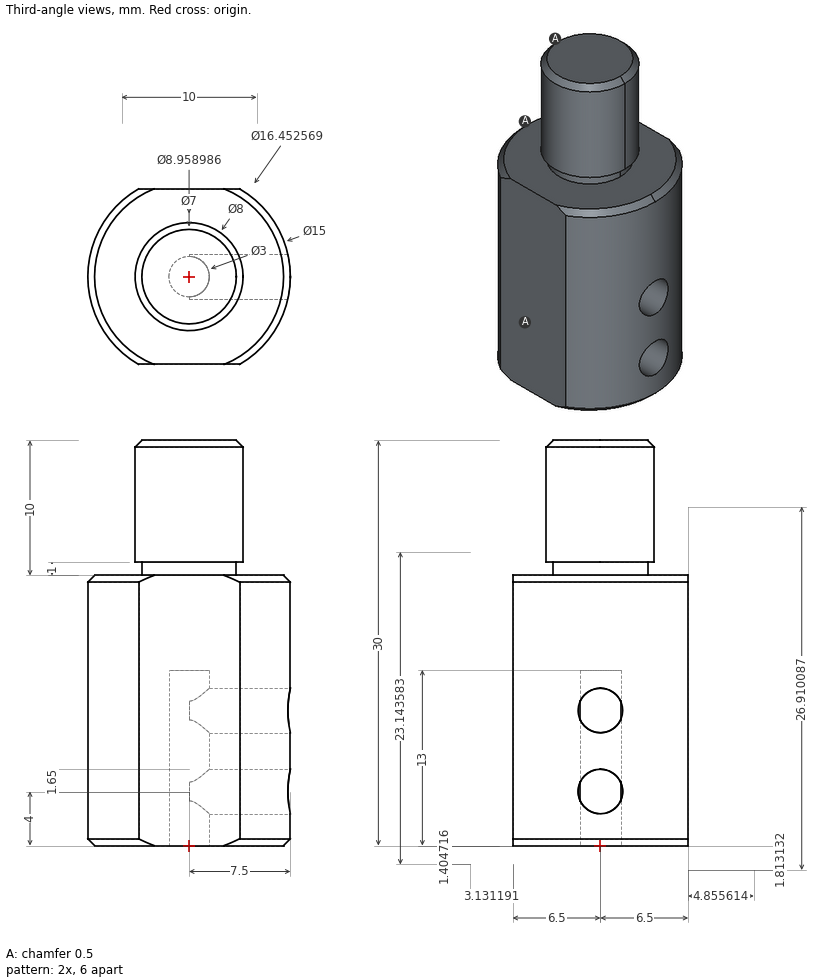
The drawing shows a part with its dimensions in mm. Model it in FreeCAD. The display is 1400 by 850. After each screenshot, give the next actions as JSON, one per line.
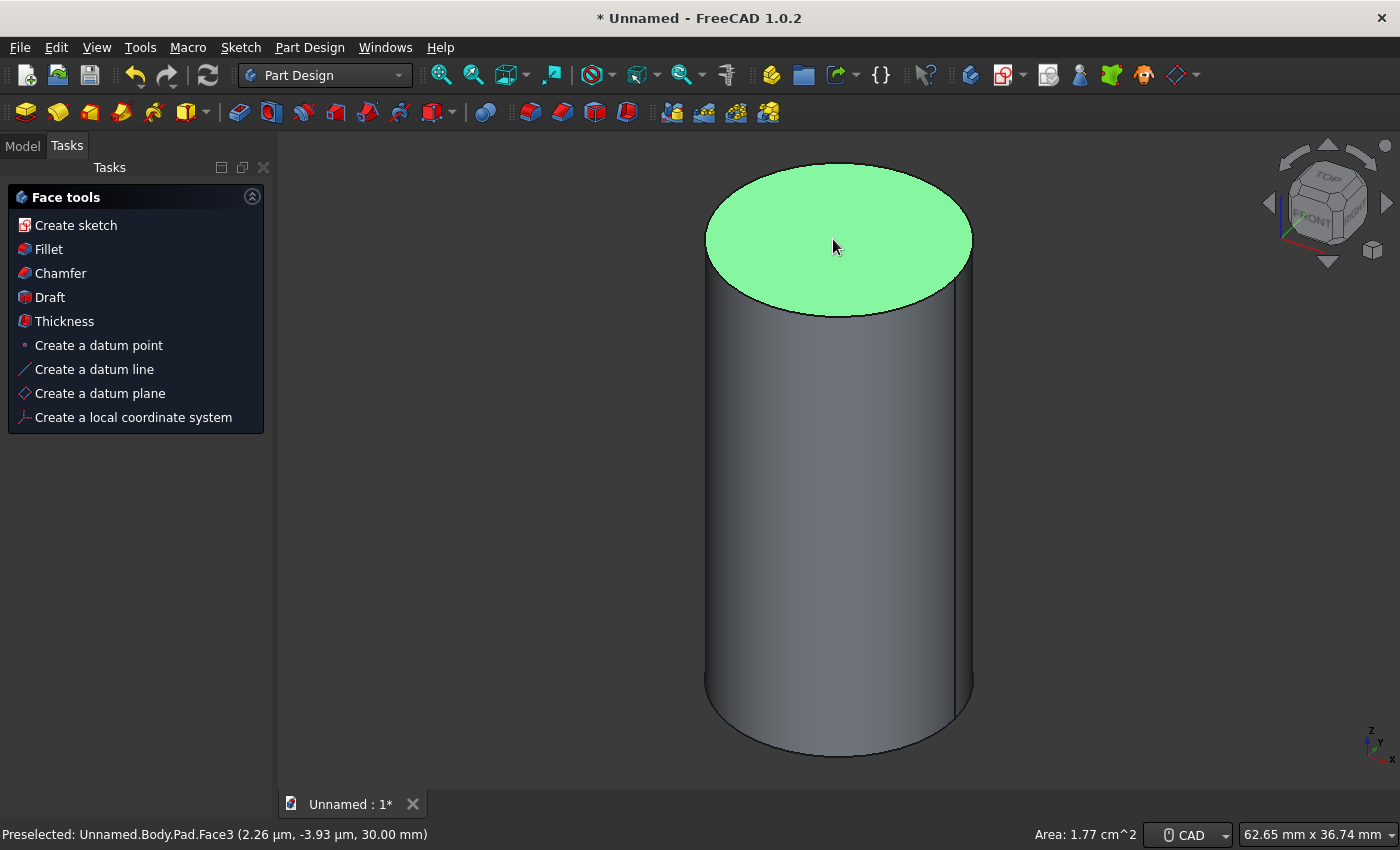
{"action": "left_click", "coordinate": [1004, 76]}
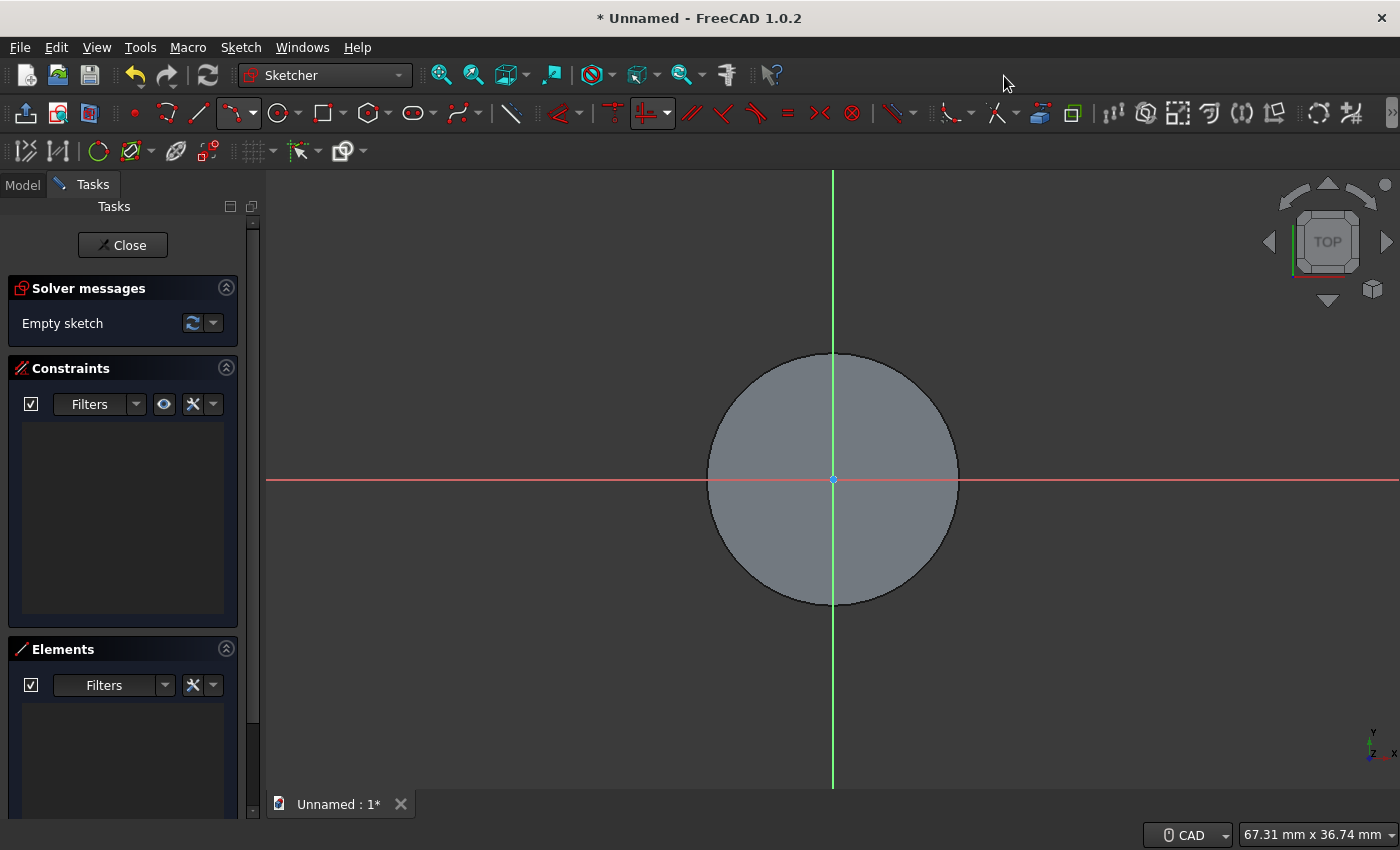
{"action": "scroll", "coordinate": [972, 480], "scroll_direction": "up", "scroll_amount": 2}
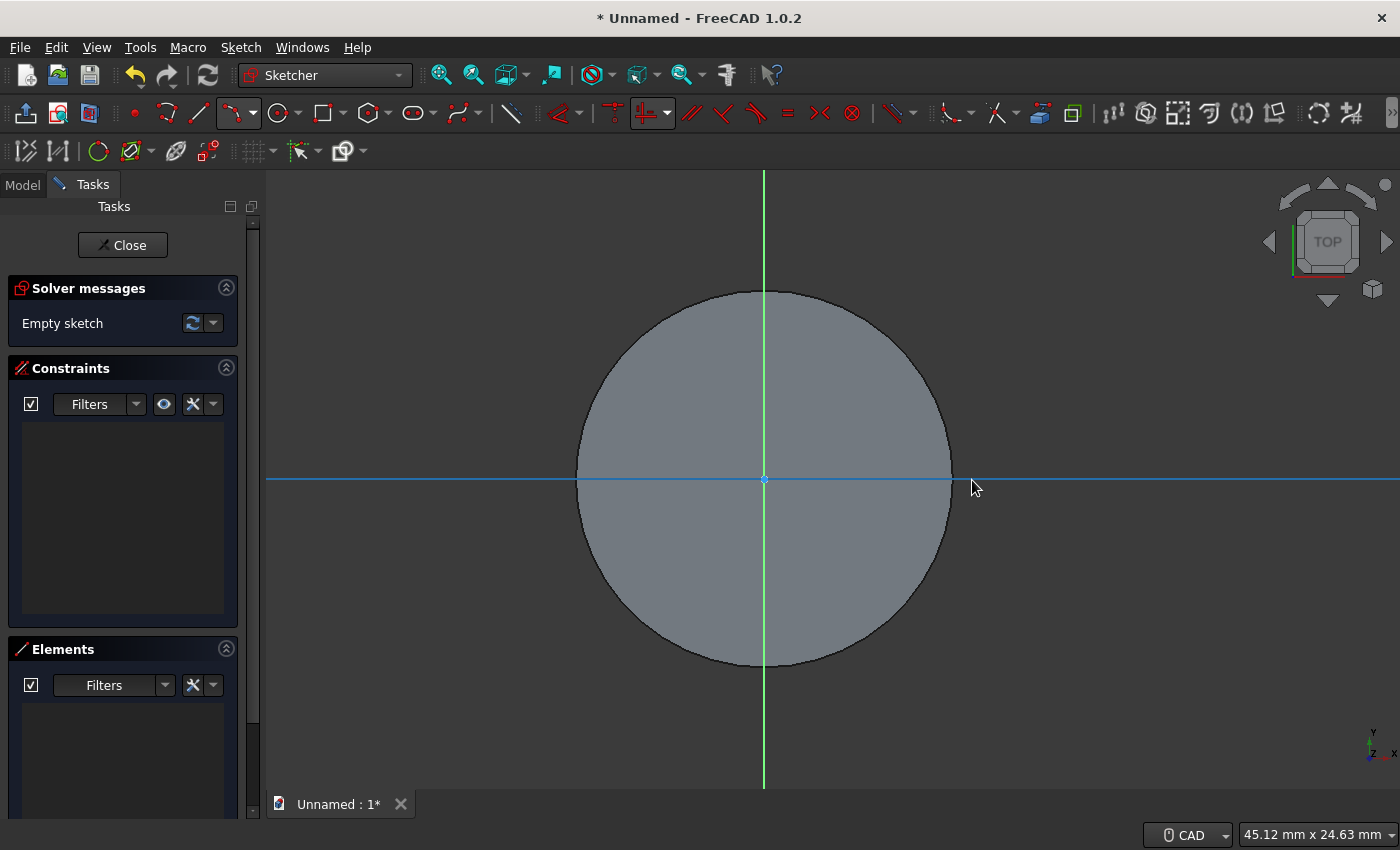
{"action": "left_click", "coordinate": [278, 114]}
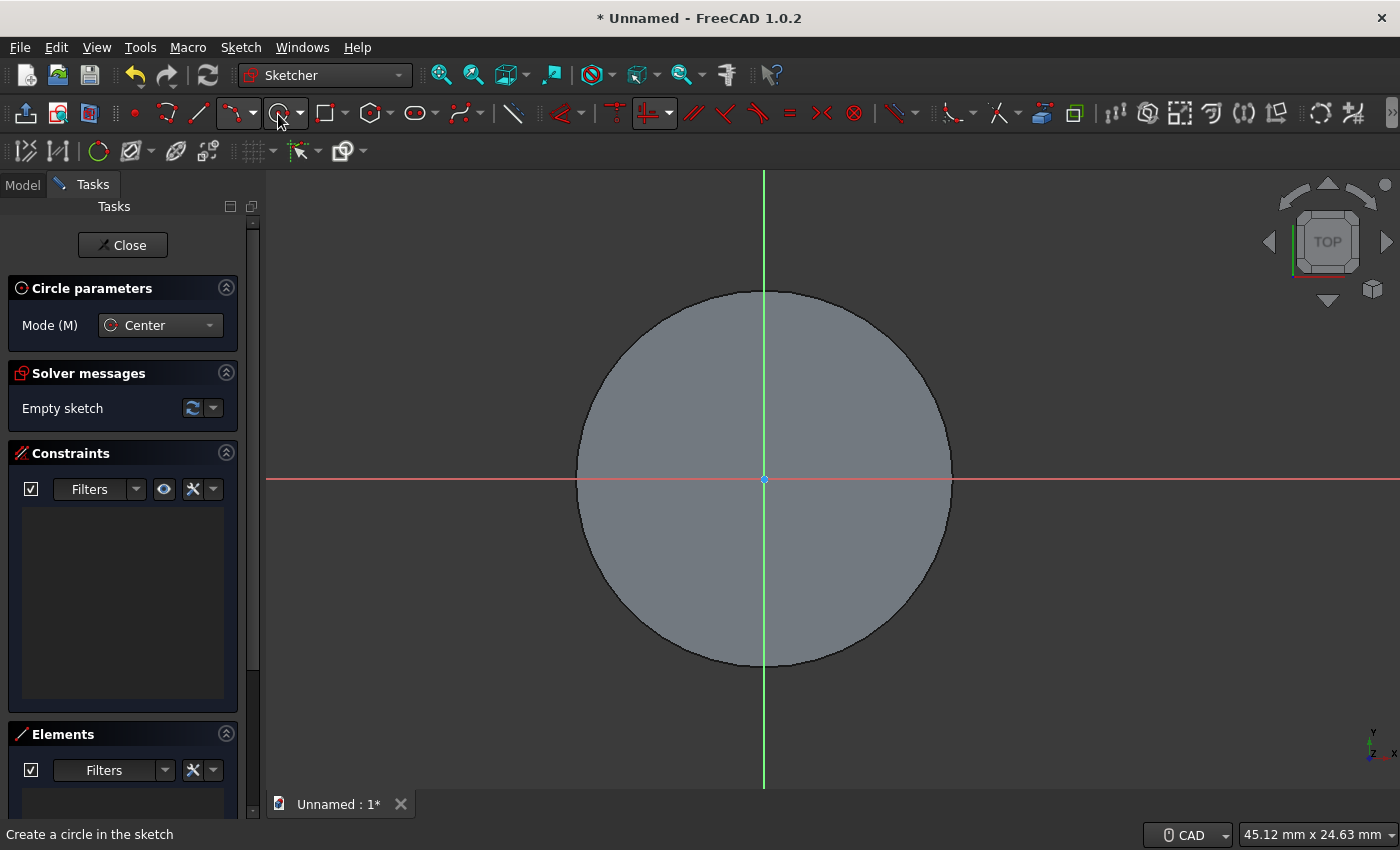
{"action": "left_click", "coordinate": [764, 479]}
{"action": "left_click", "coordinate": [911, 333]}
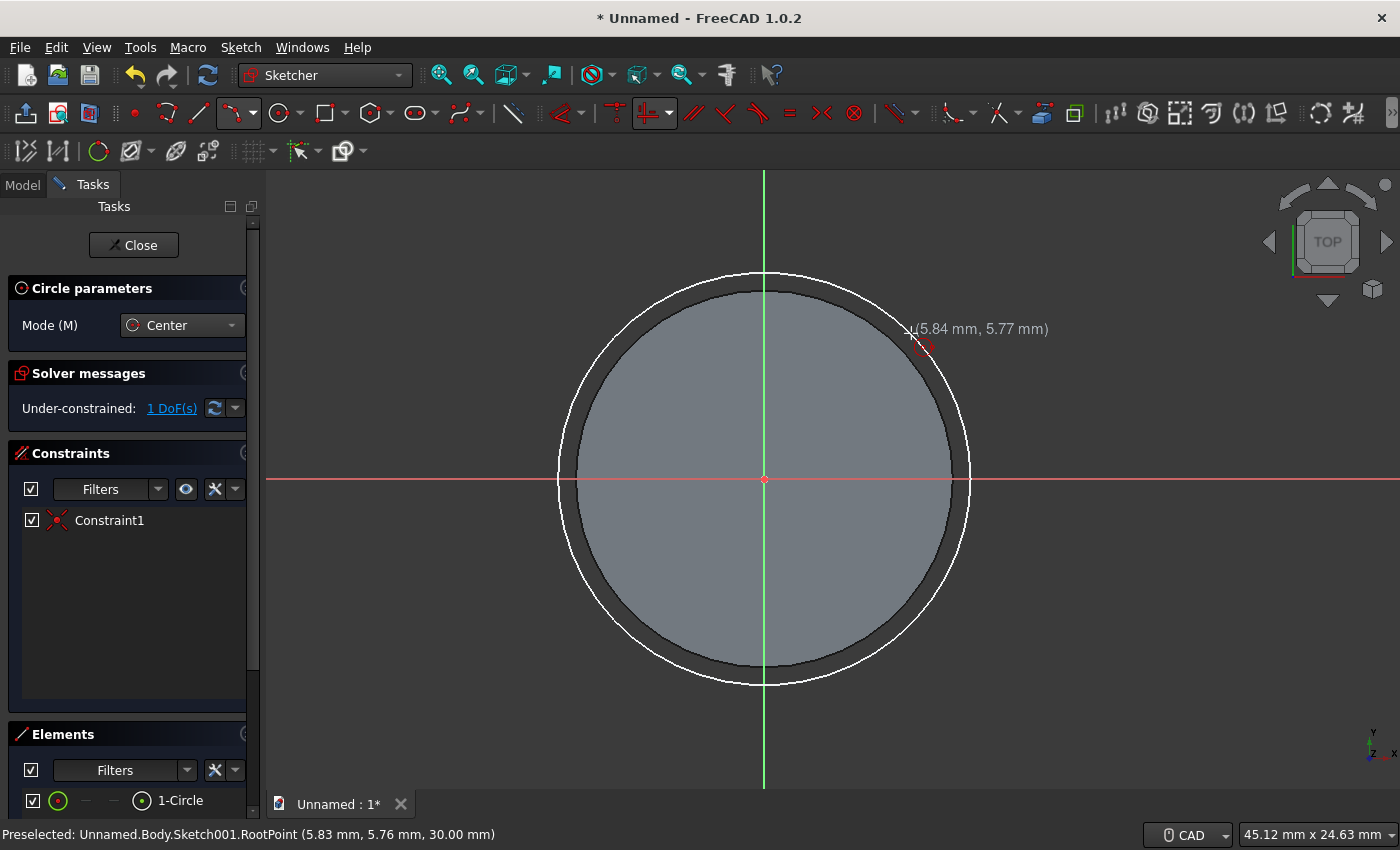
{"action": "left_click", "coordinate": [764, 479]}
{"action": "left_click", "coordinate": [835, 408]}
{"action": "key", "text": "Escape"}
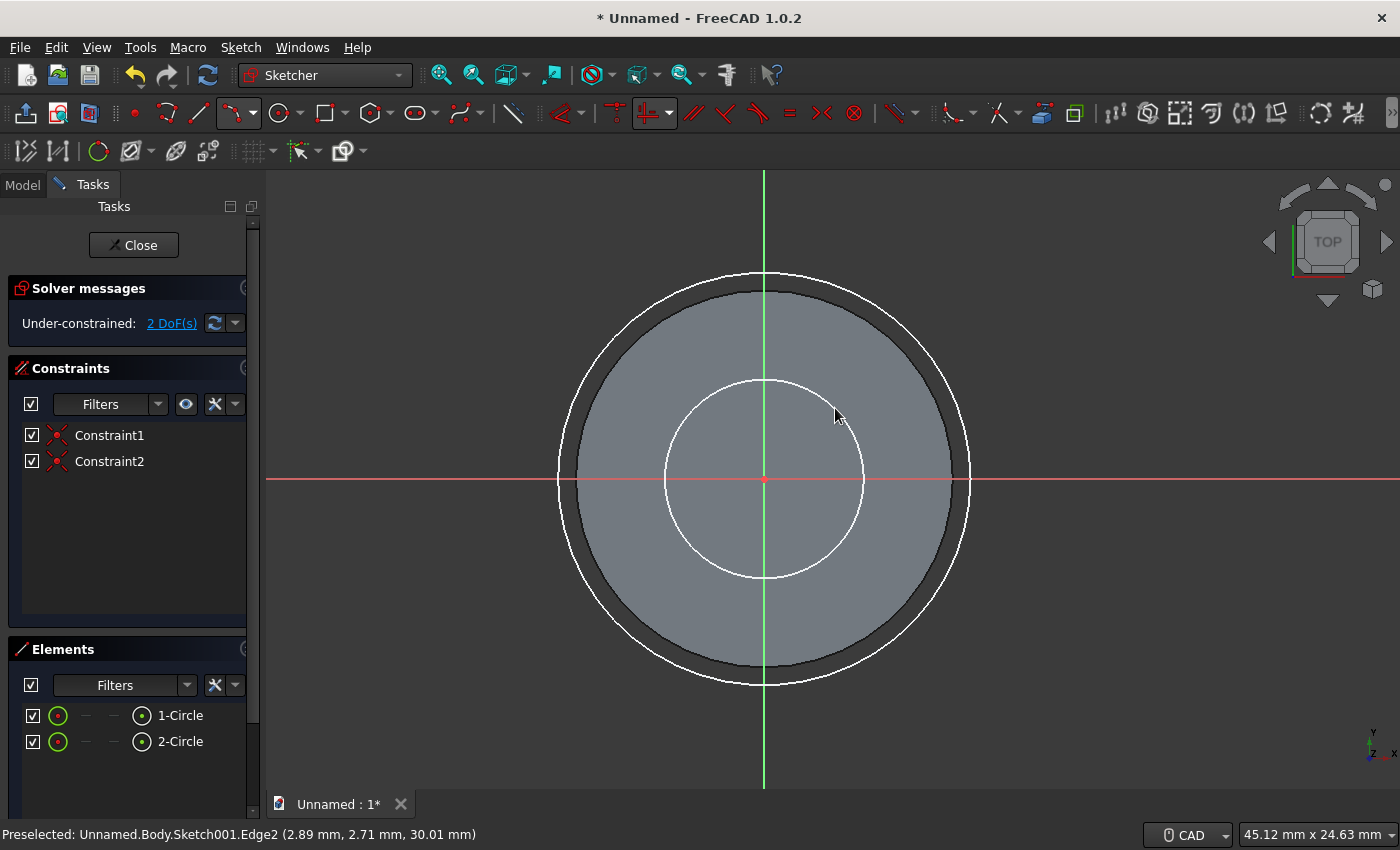
{"action": "left_click", "coordinate": [560, 114]}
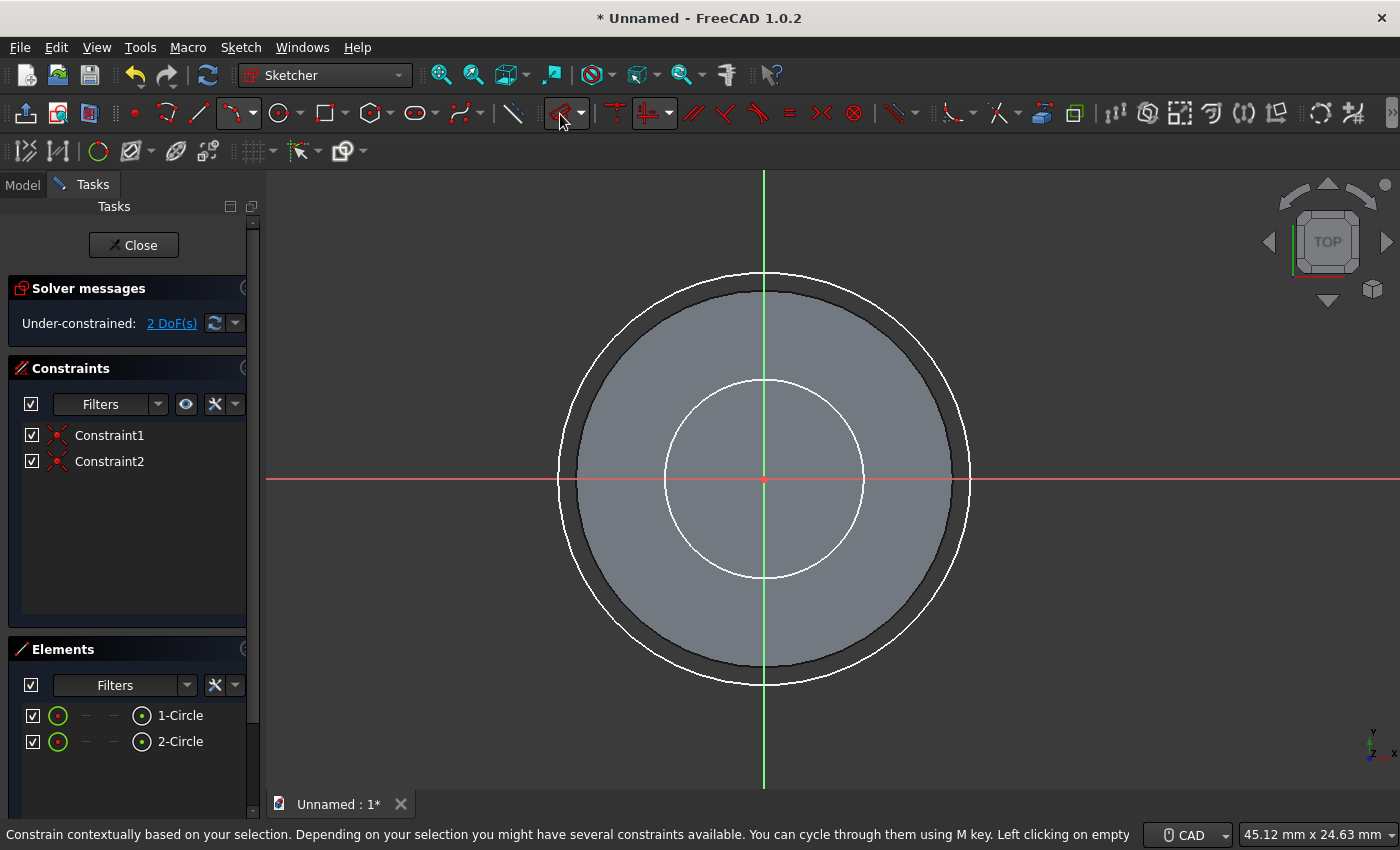
{"action": "left_click", "coordinate": [910, 333]}
{"action": "left_click", "coordinate": [933, 310]}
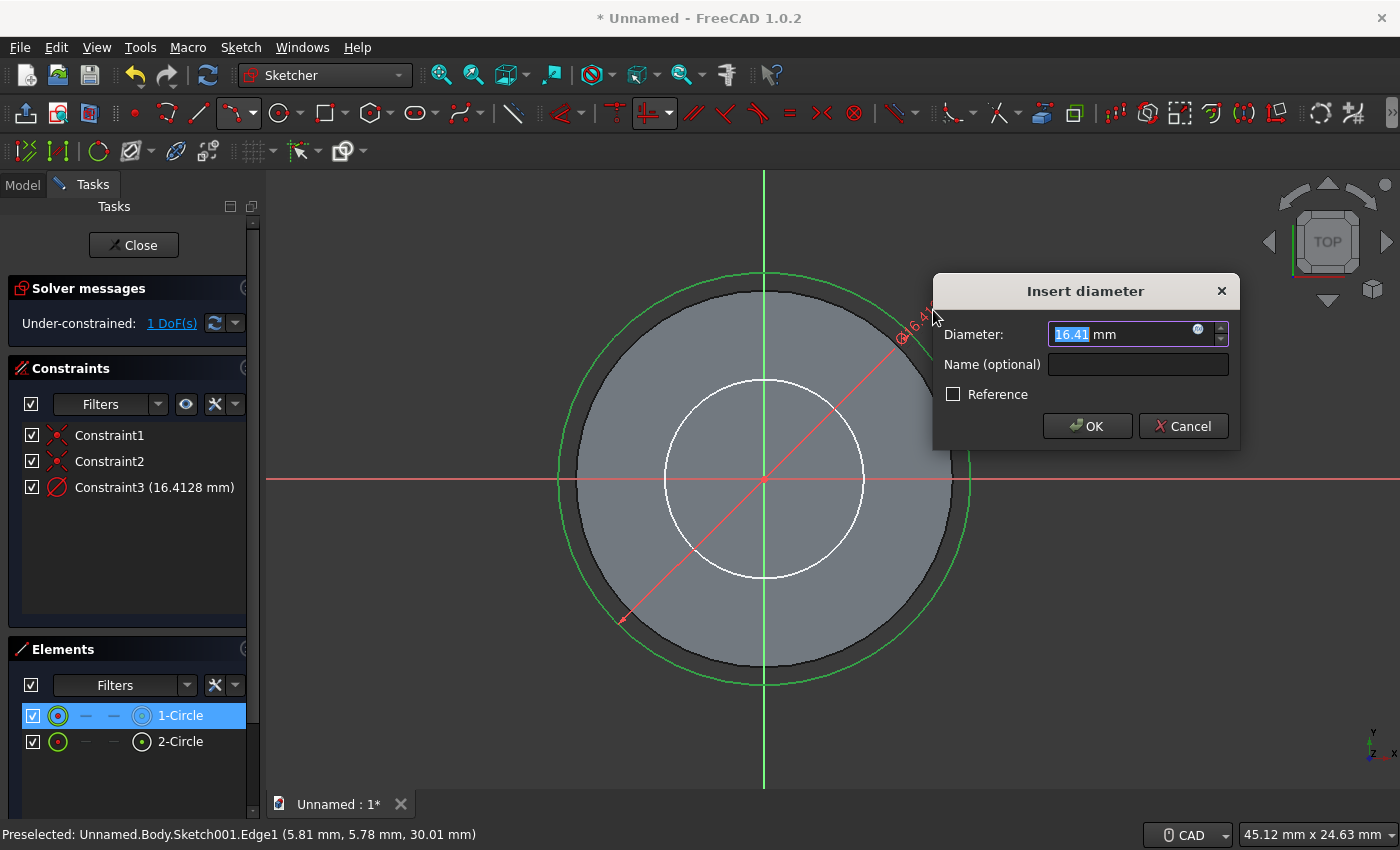
{"action": "type", "text": "16.452569"}
{"action": "key", "text": "Return"}